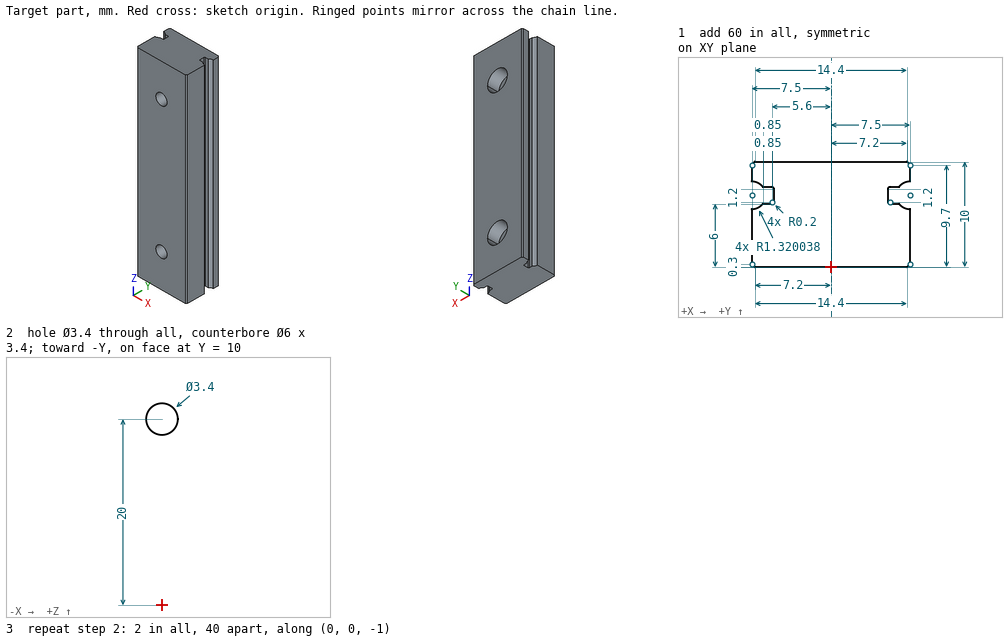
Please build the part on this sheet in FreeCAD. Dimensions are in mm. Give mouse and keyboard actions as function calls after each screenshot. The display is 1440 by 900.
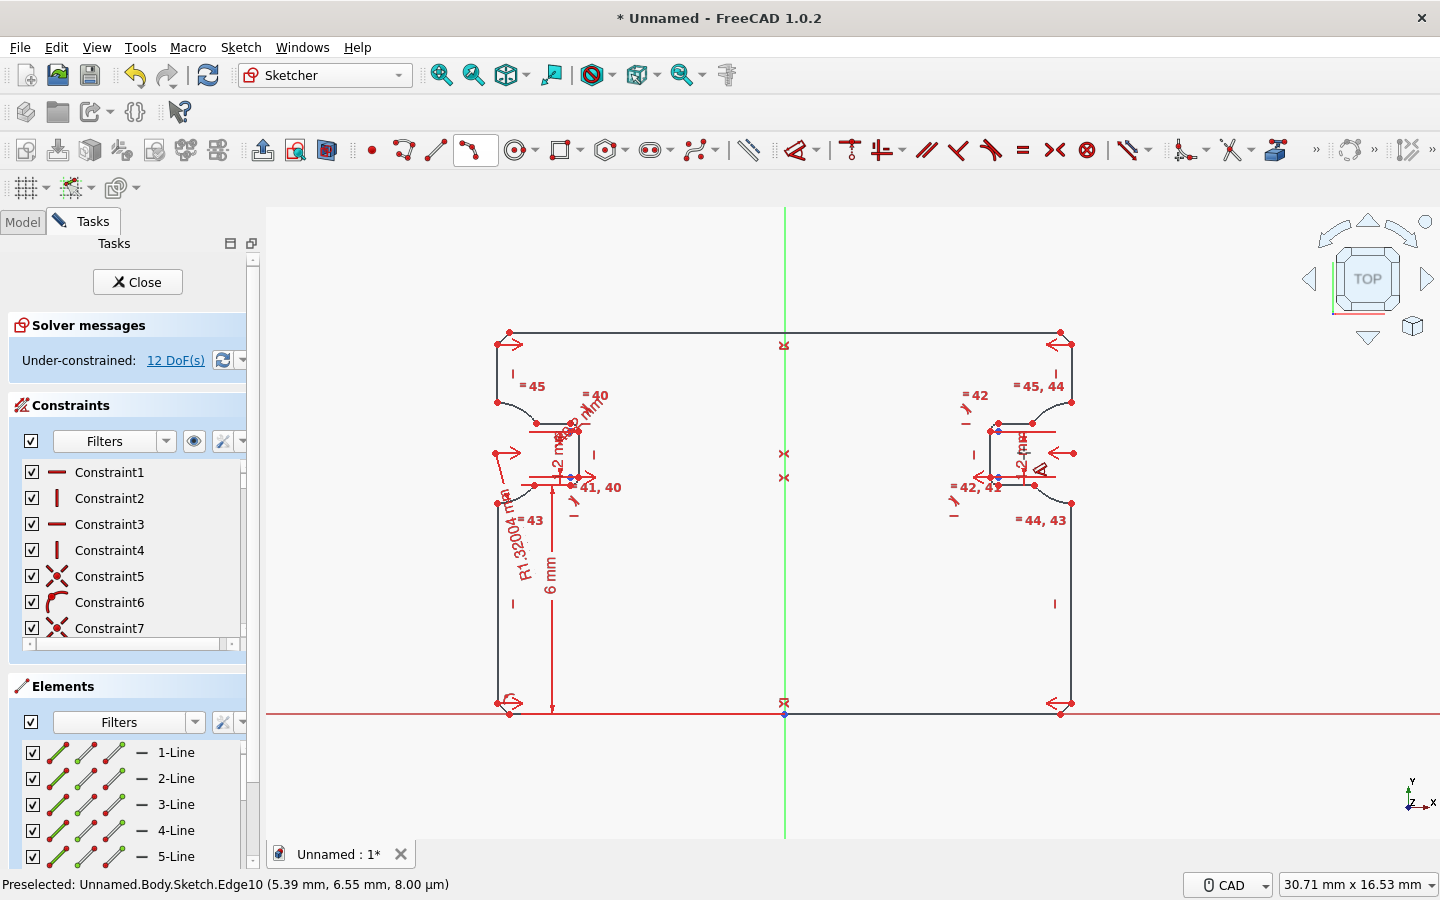
click(1060, 333)
click(1094, 524)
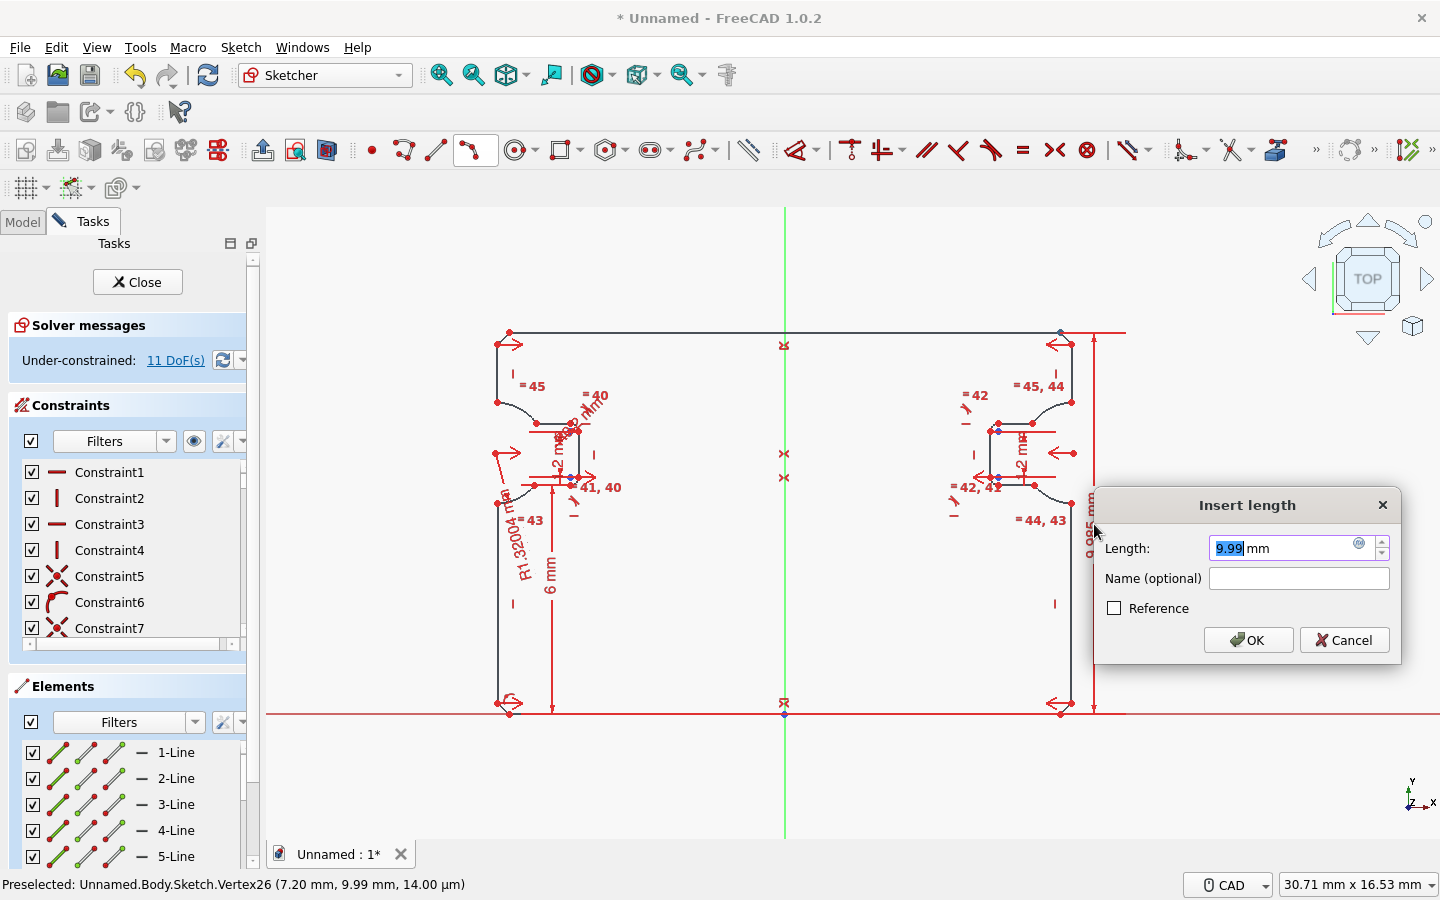
text(10)
key(Return)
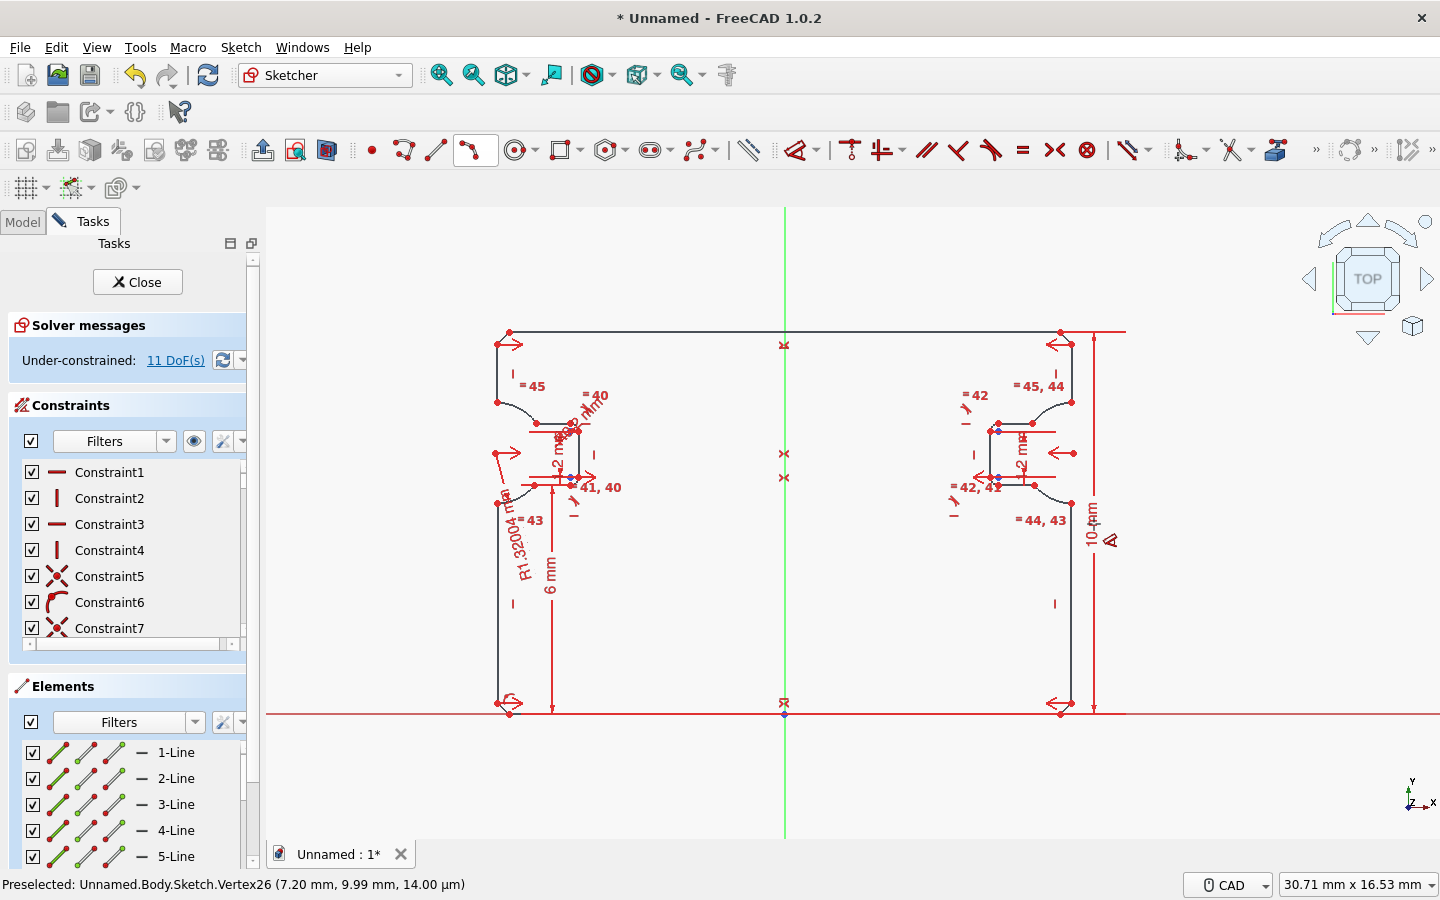
scroll(547, 424, up, 2)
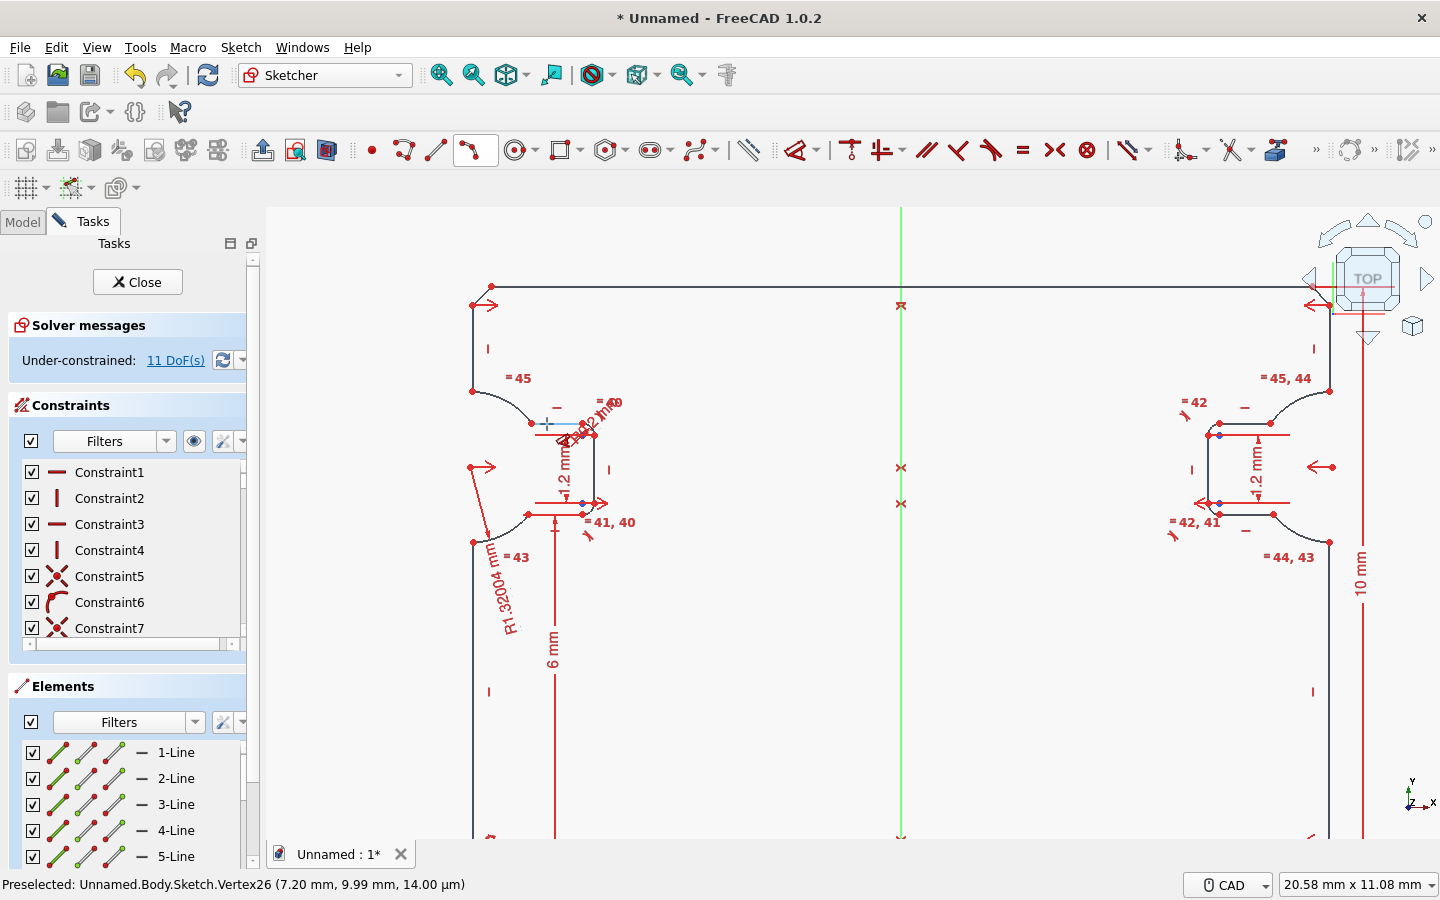
click(547, 424)
click(557, 390)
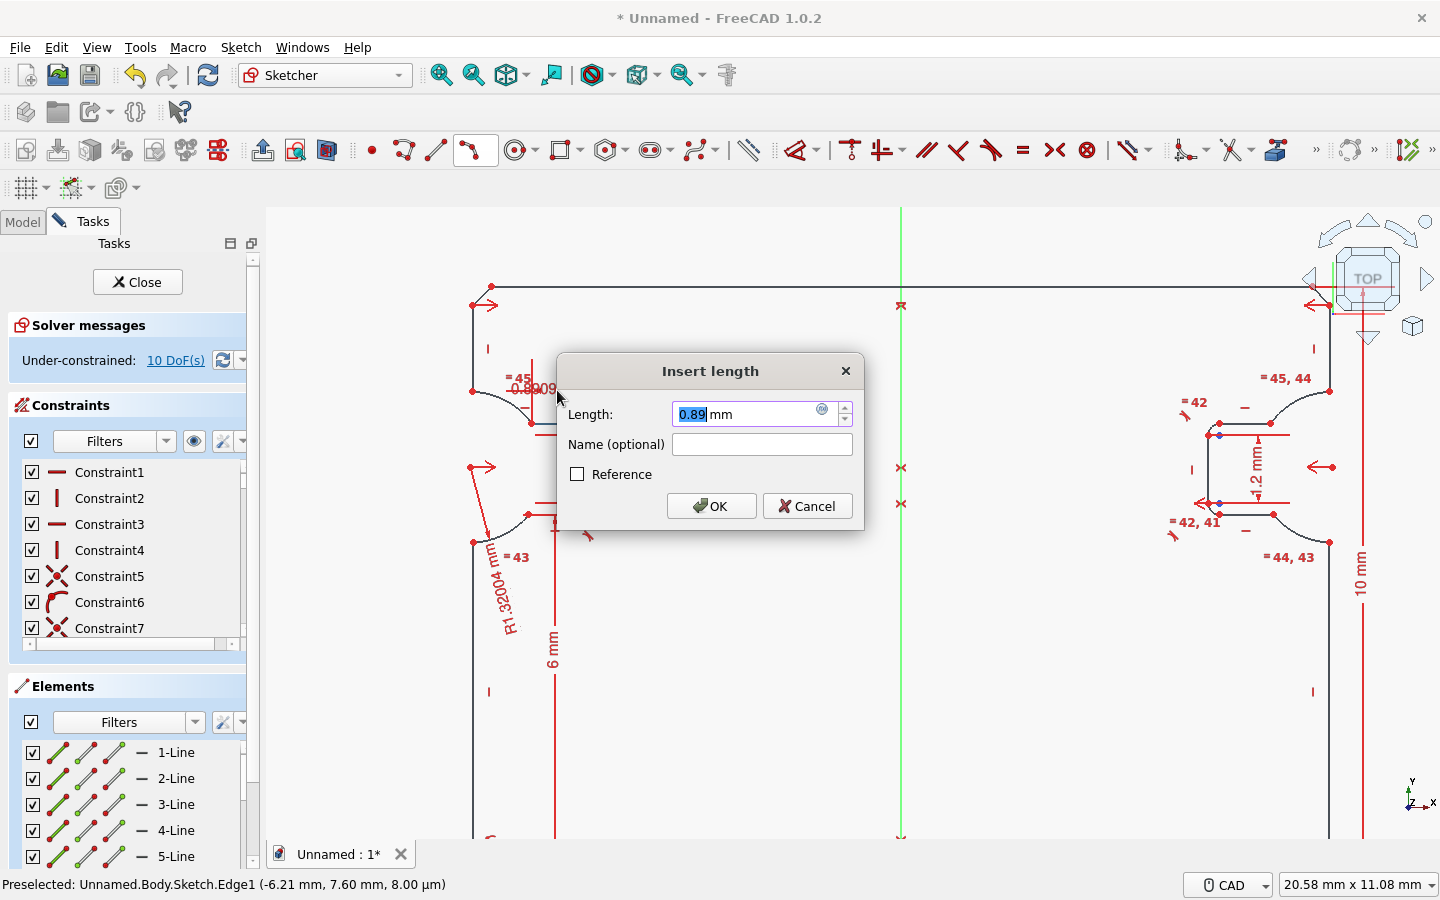
text(0.85)
key(Return)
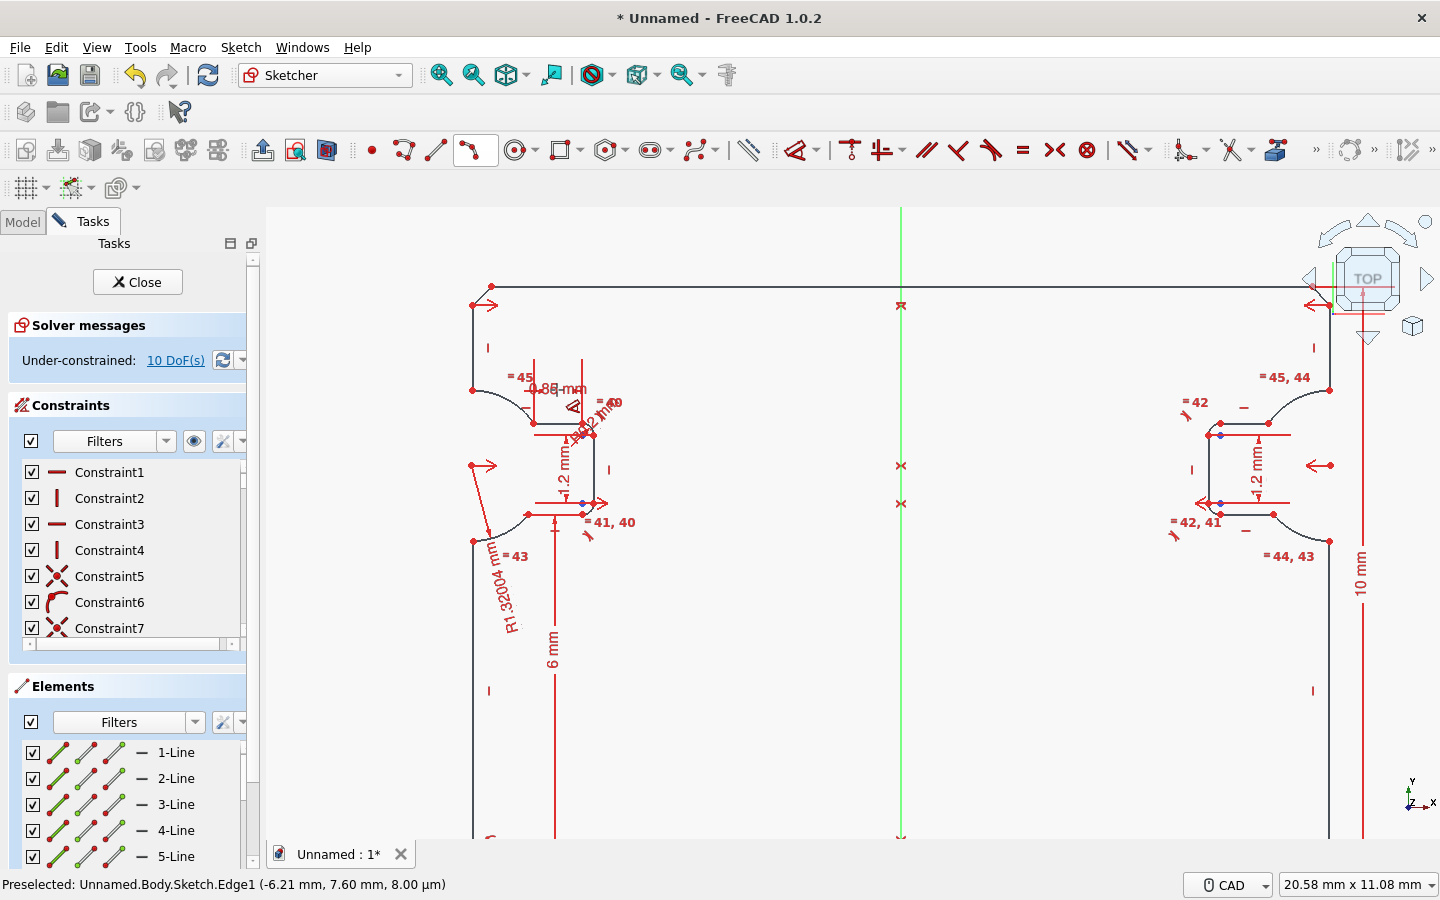
click(566, 515)
click(556, 549)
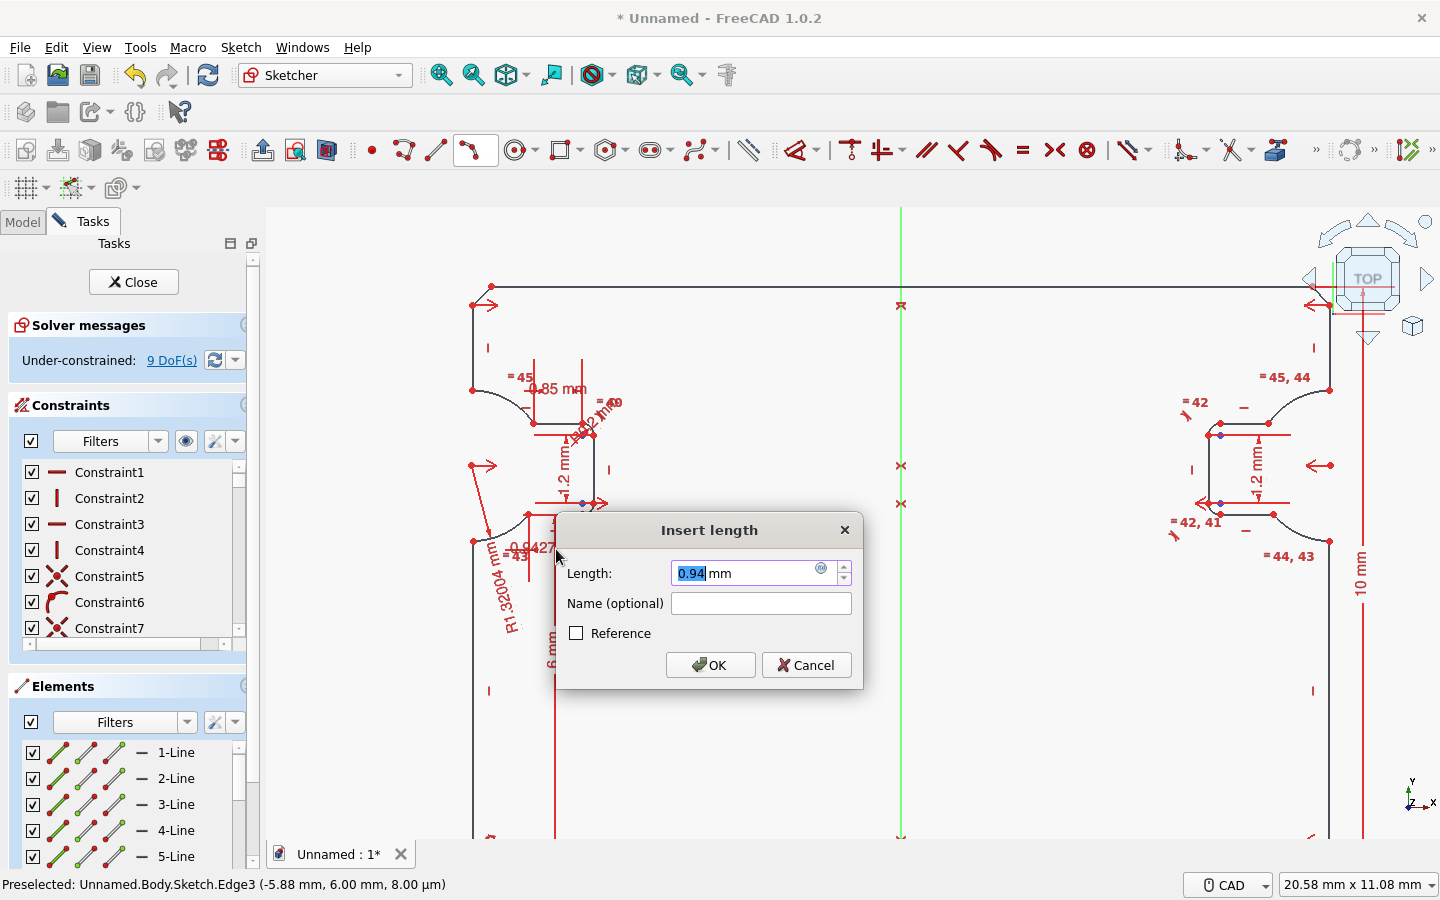
text(0.85)
key(Return)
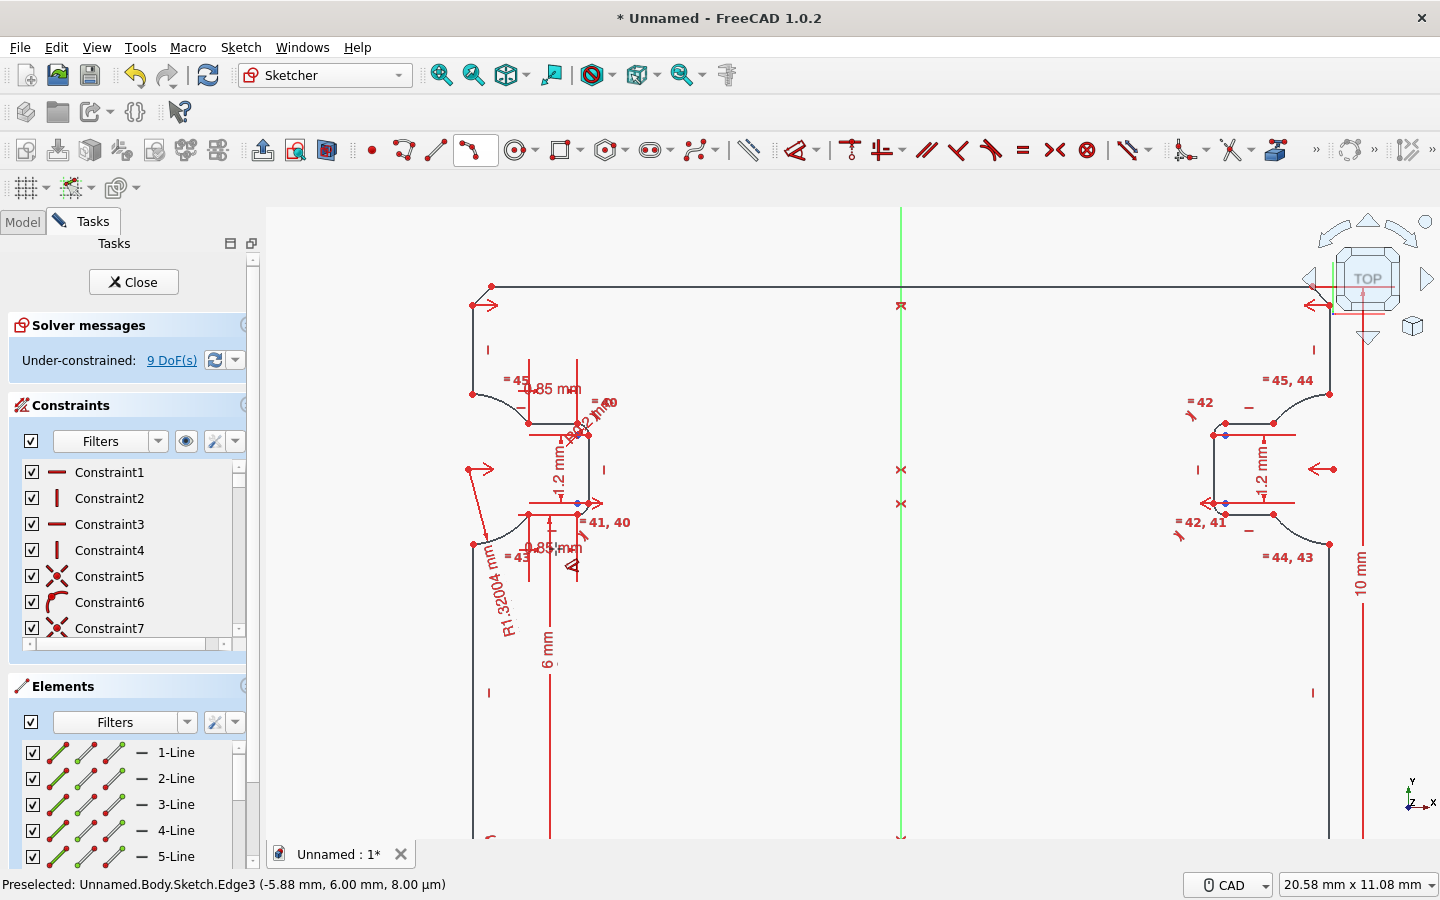
scroll(547, 423, down, 2)